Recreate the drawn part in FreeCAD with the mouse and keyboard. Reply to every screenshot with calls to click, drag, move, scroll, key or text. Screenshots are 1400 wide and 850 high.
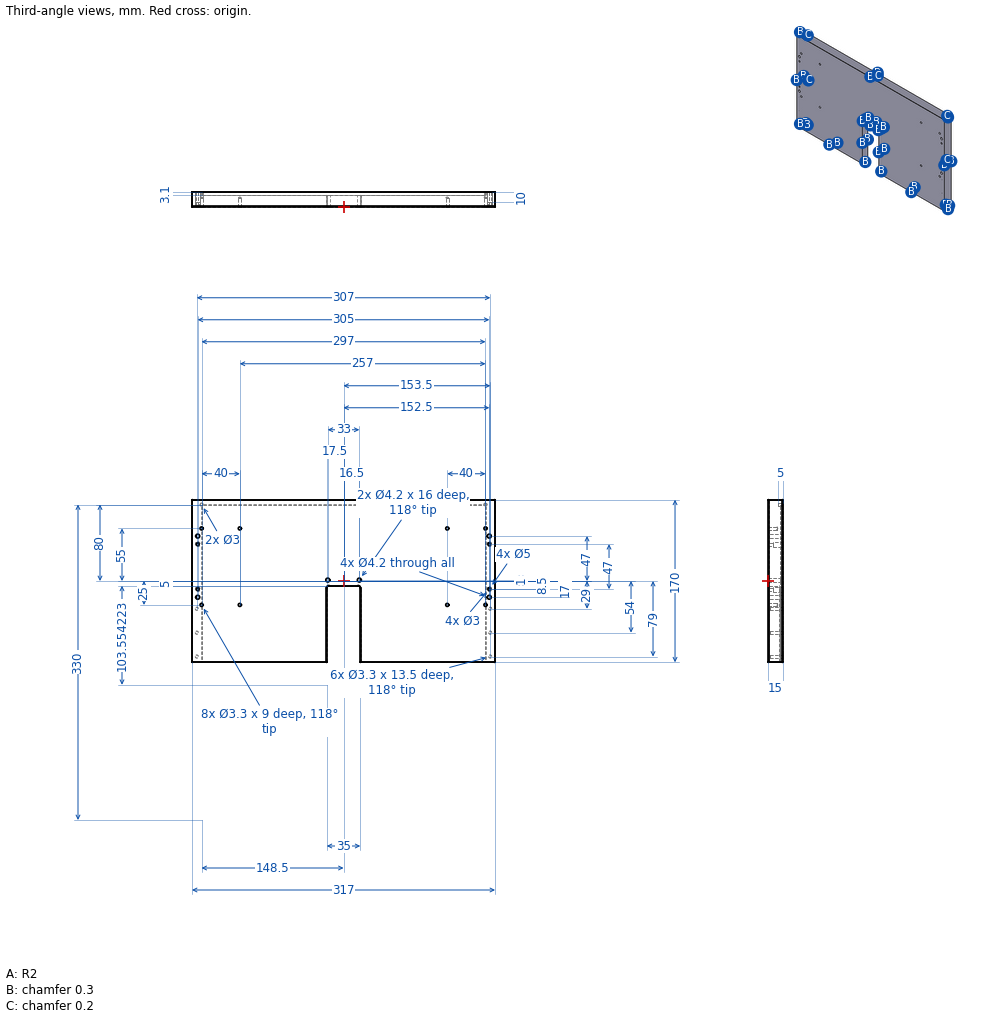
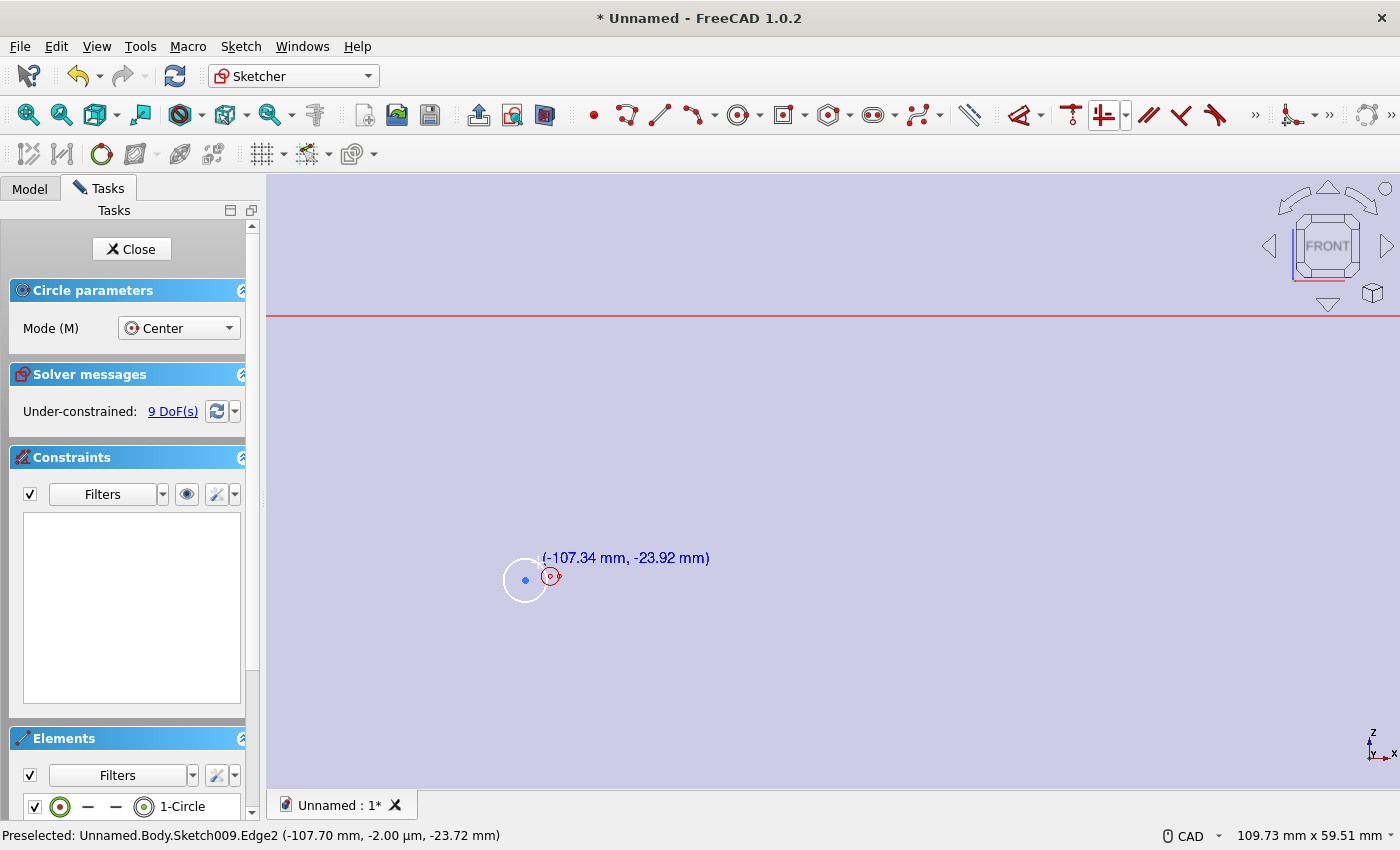
scroll(541, 563, down, 8)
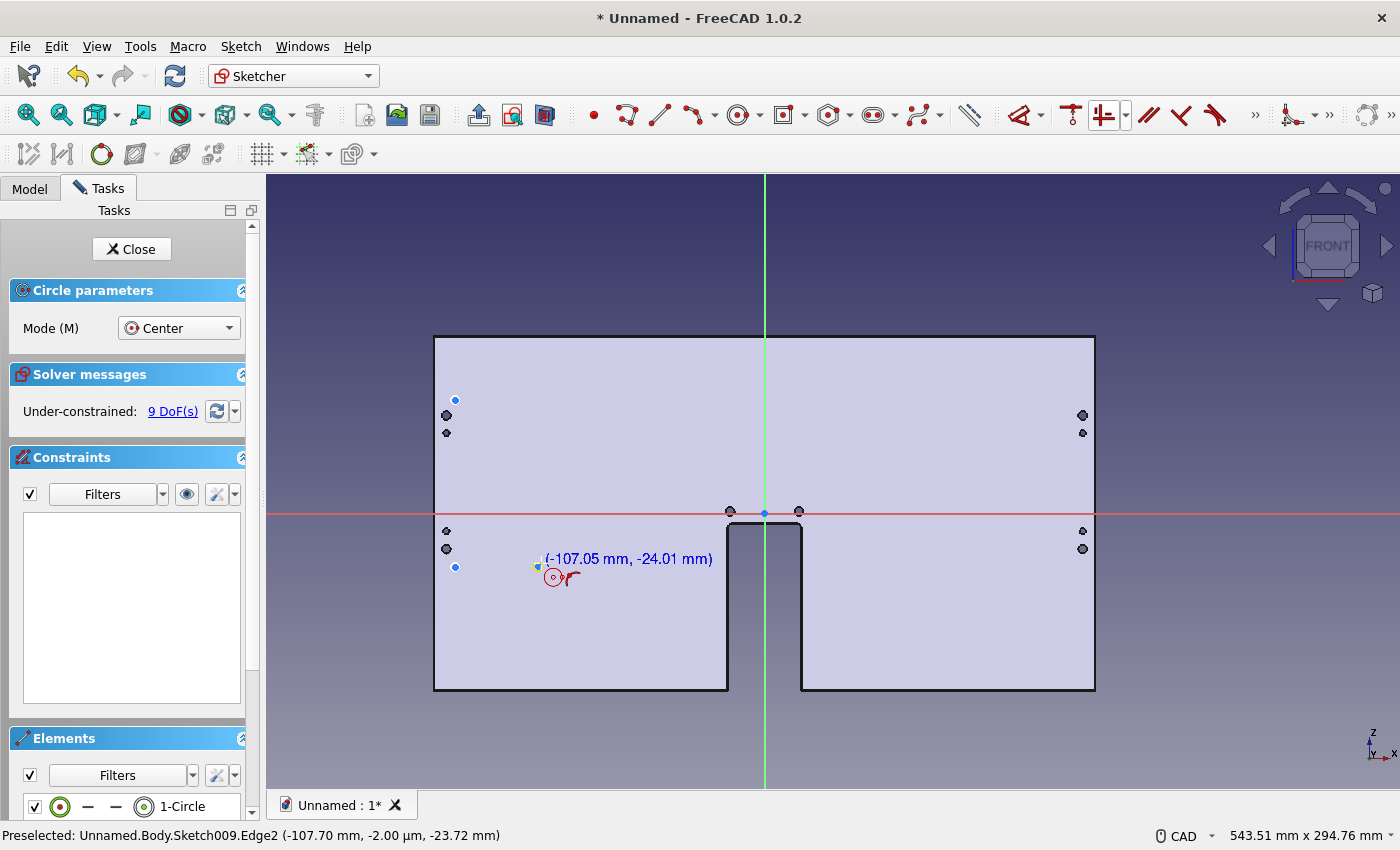
scroll(538, 399, up, 10)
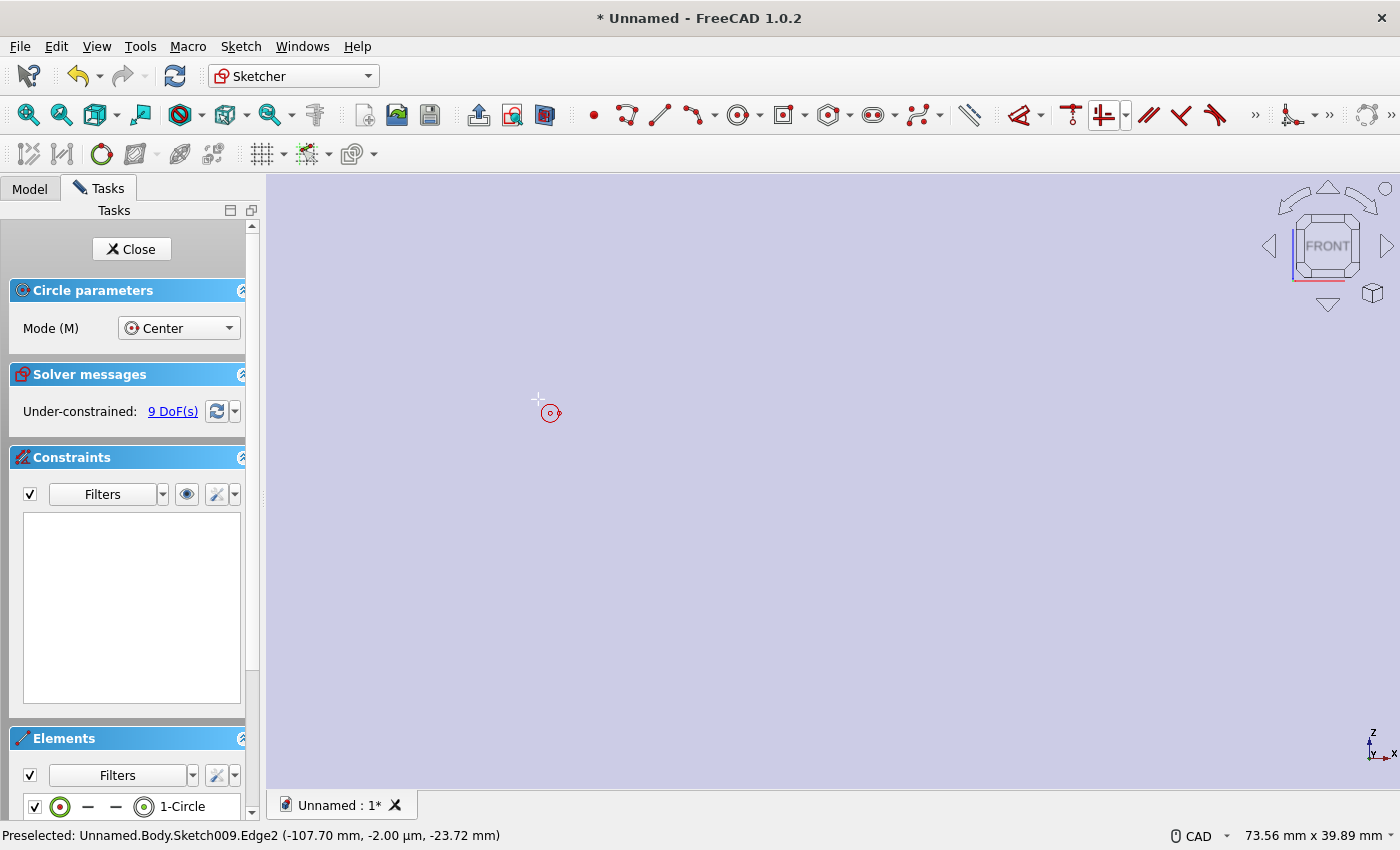
scroll(538, 398, down, 10)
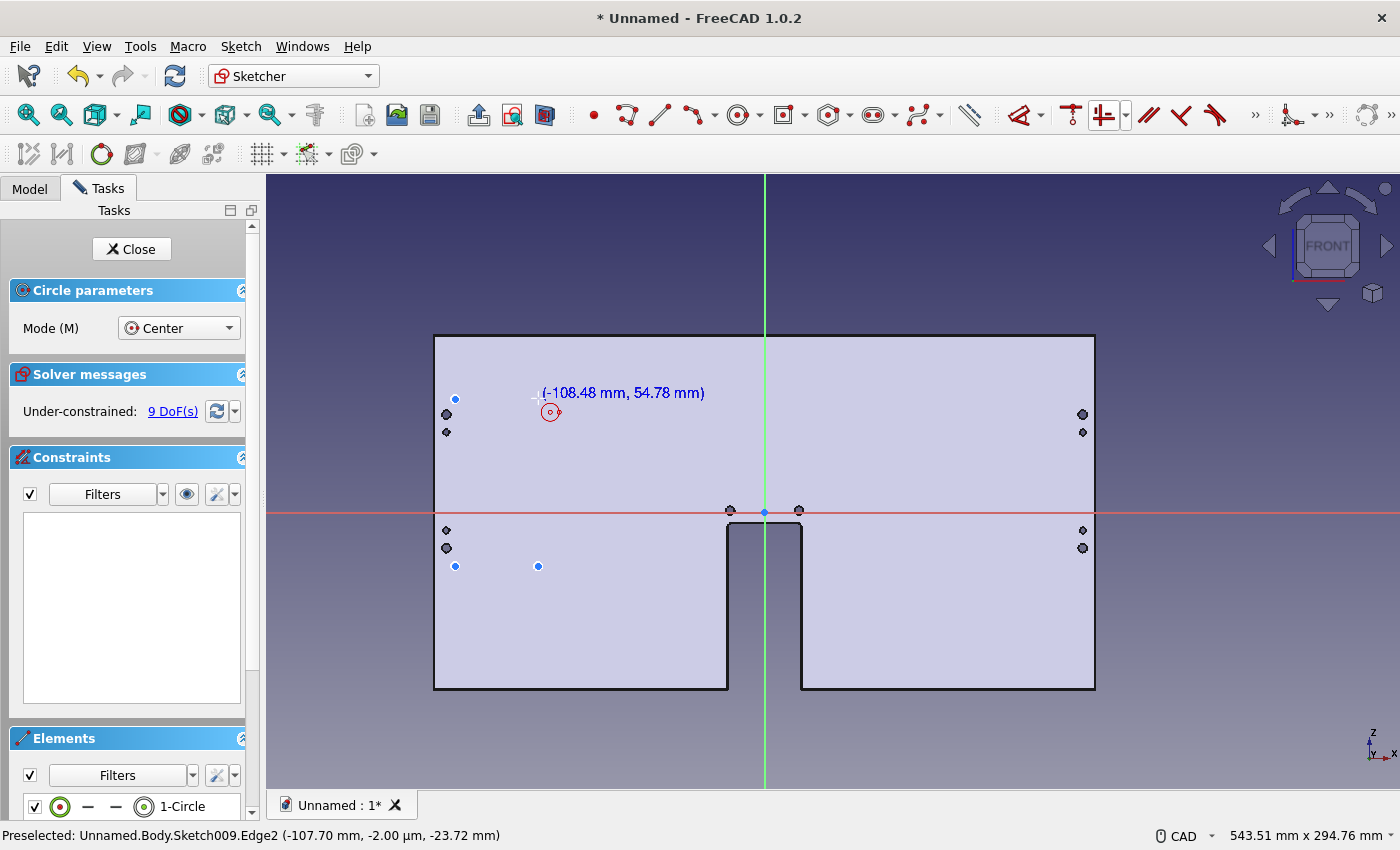
click(538, 398)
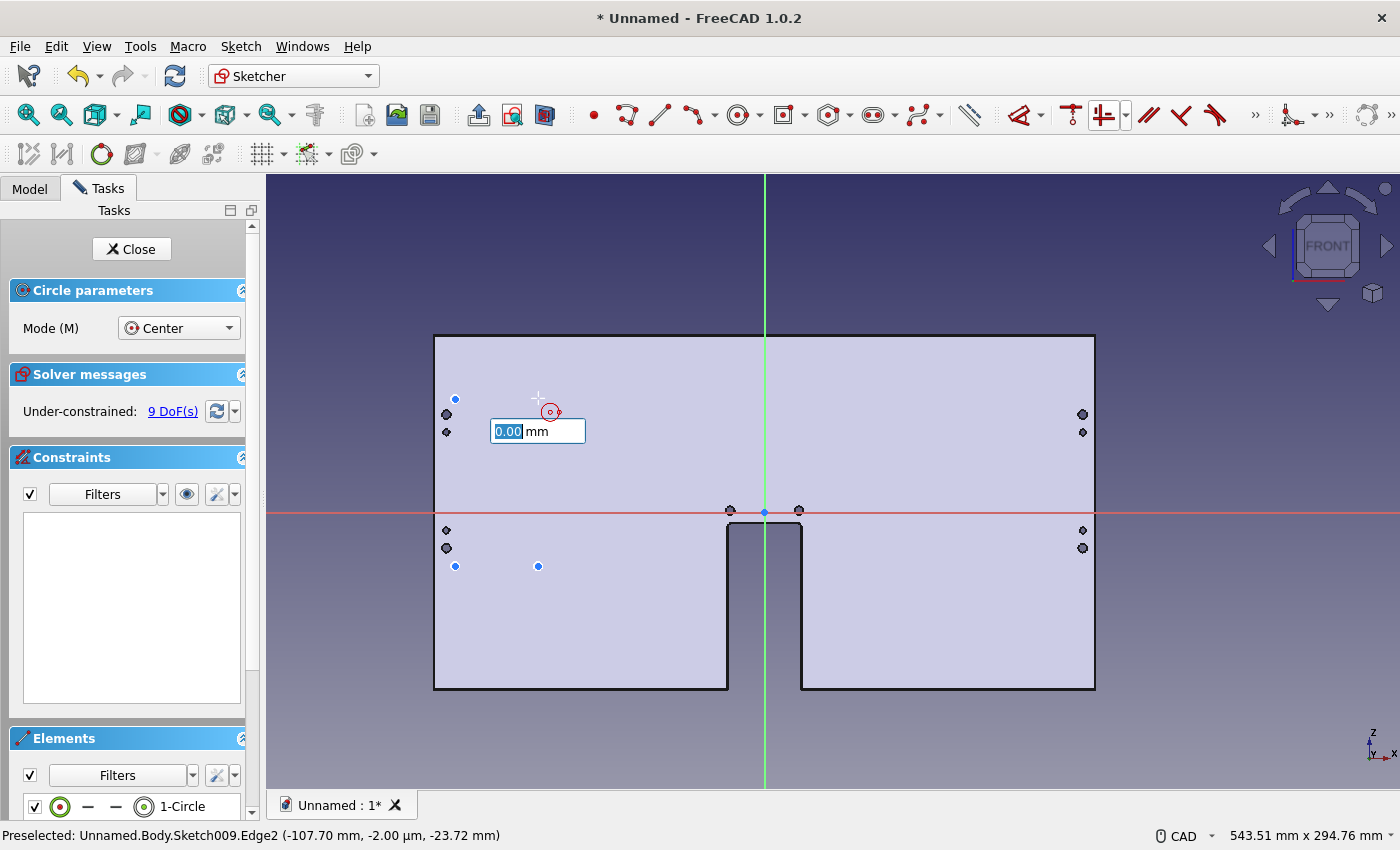
scroll(541, 396, up, 8)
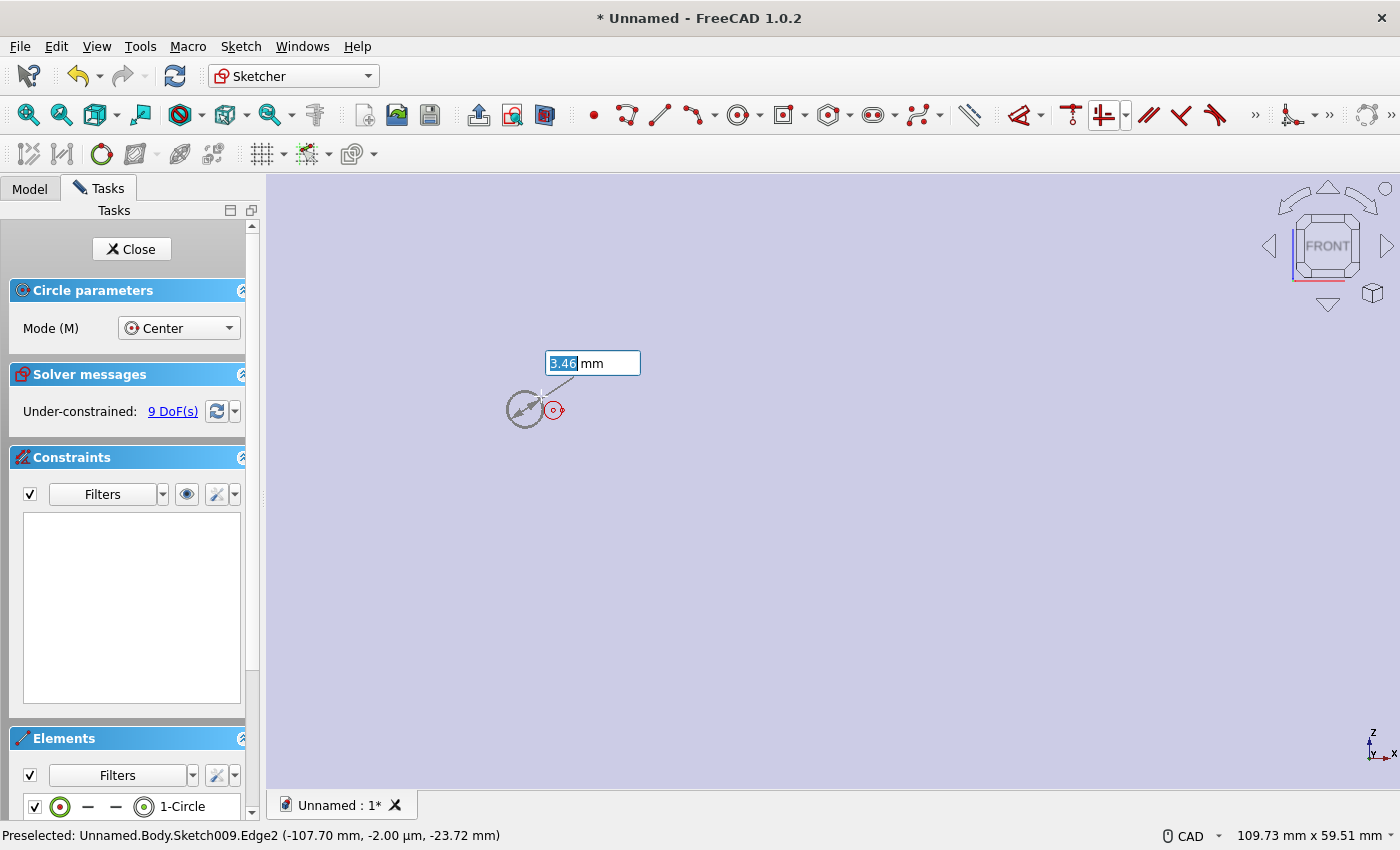
click(538, 392)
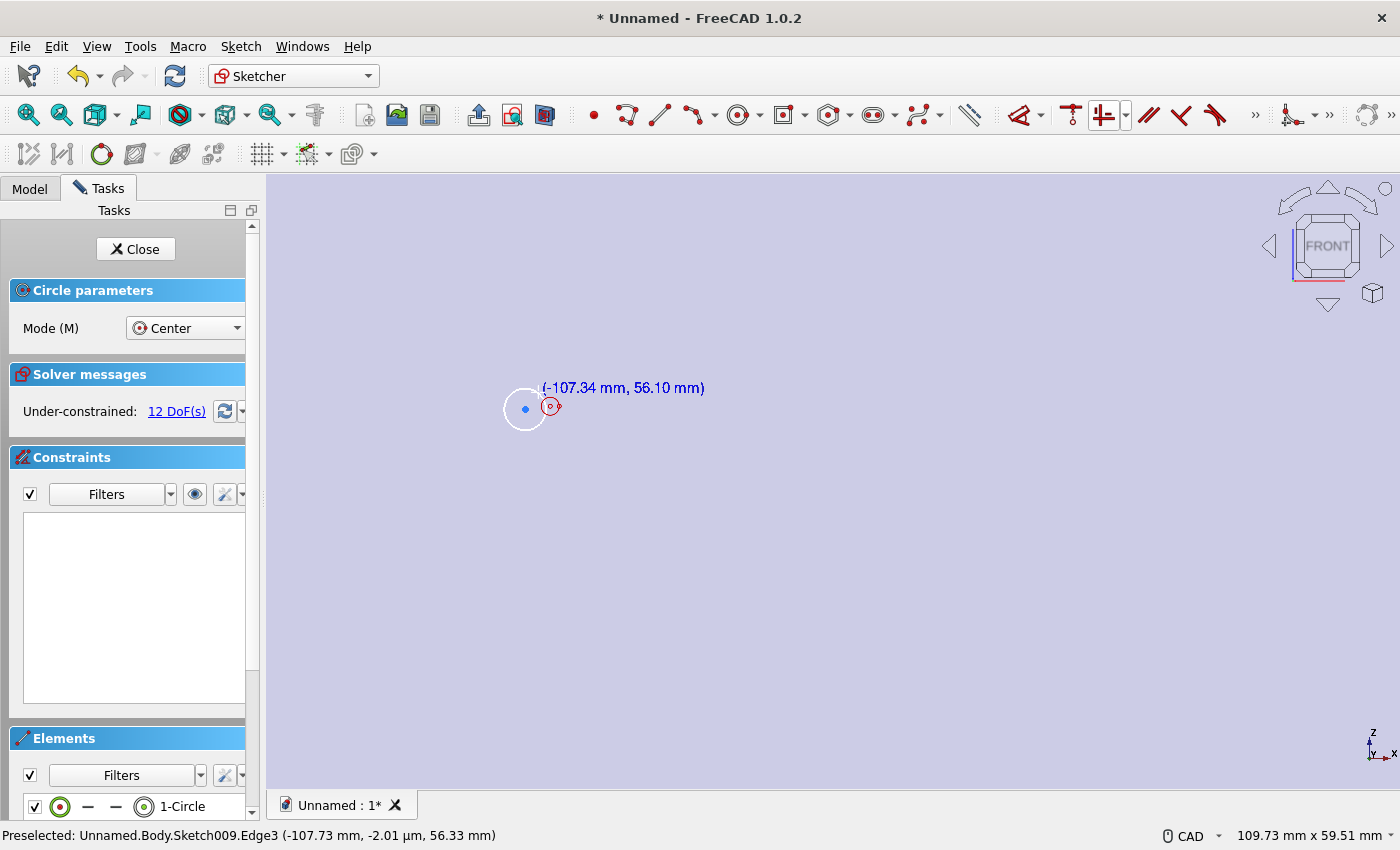
scroll(541, 396, down, 8)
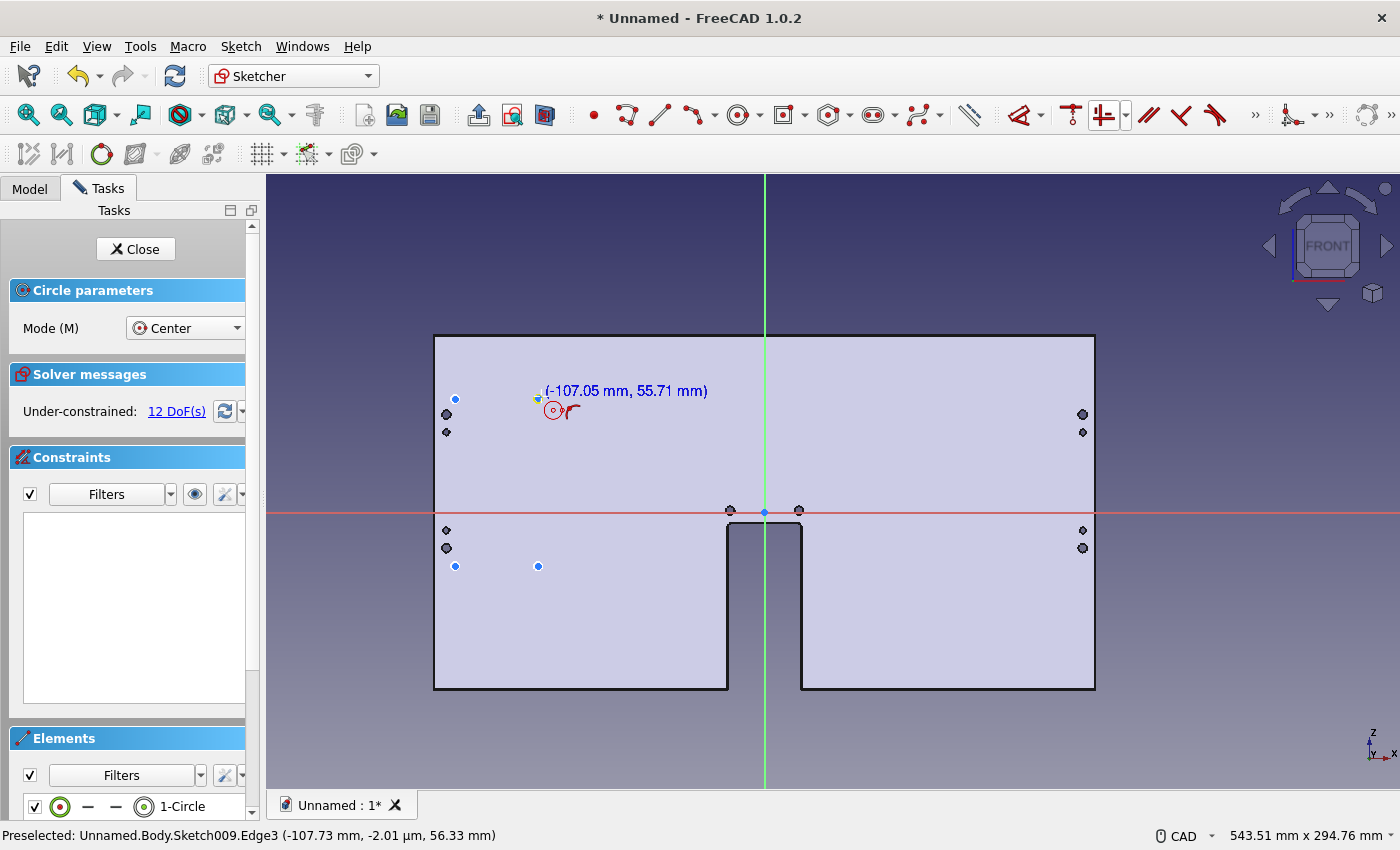
scroll(1074, 565, up, 10)